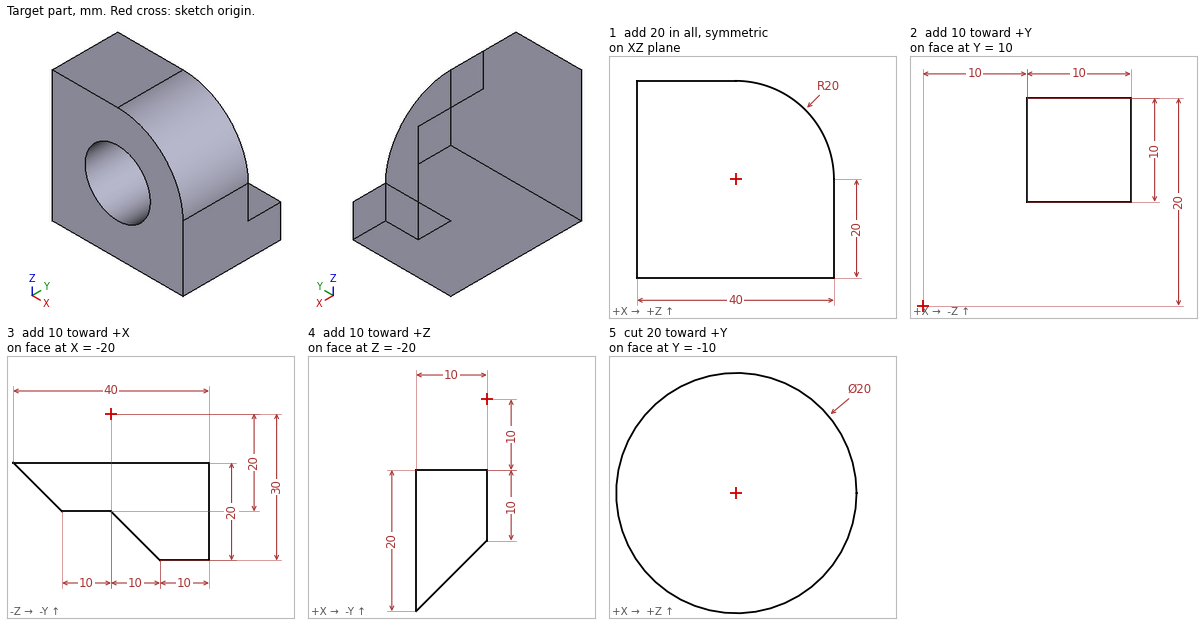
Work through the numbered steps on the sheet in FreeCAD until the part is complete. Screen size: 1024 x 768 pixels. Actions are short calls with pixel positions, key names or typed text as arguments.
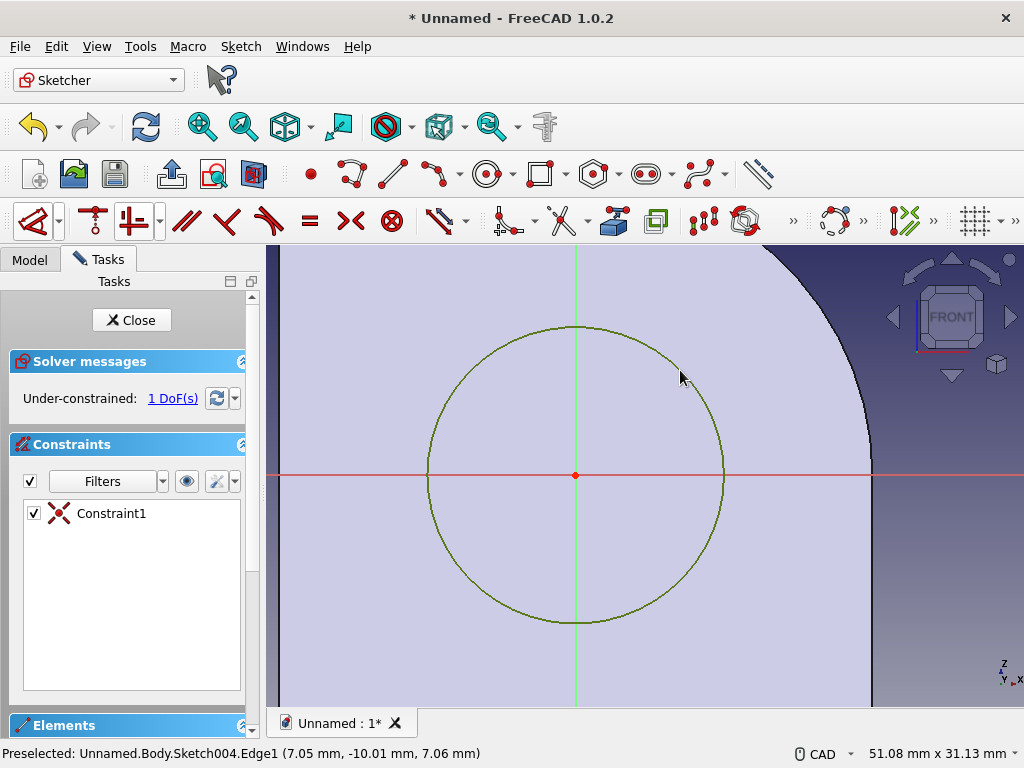
key(k)
key(o)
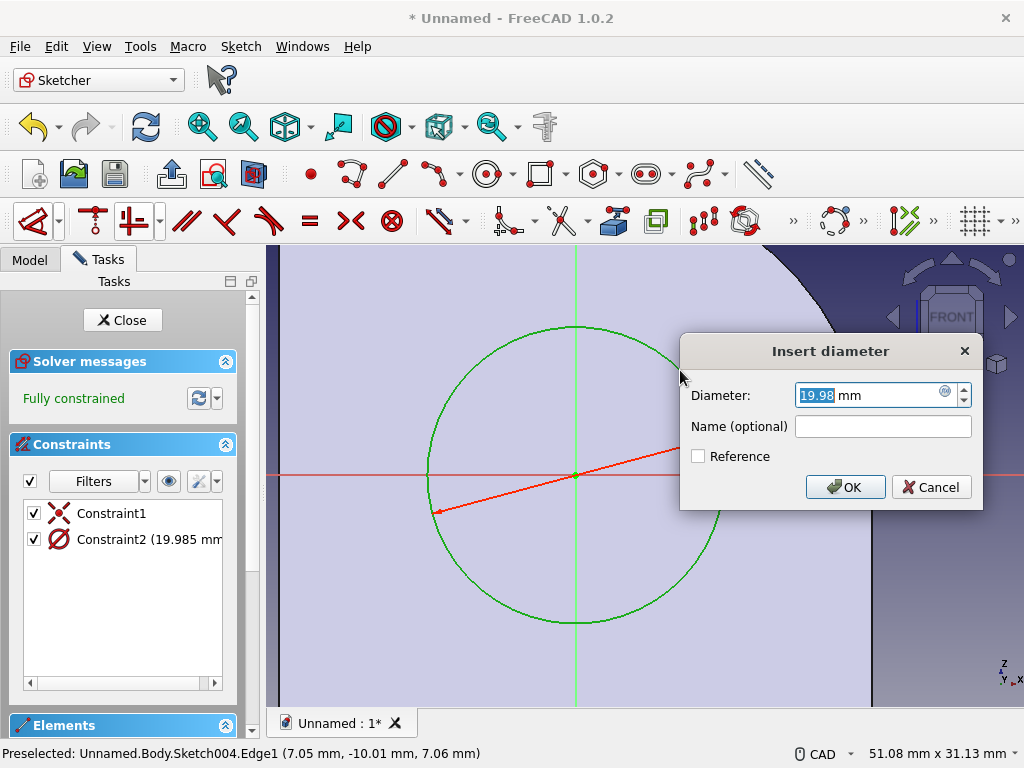
text(20)
key(Return)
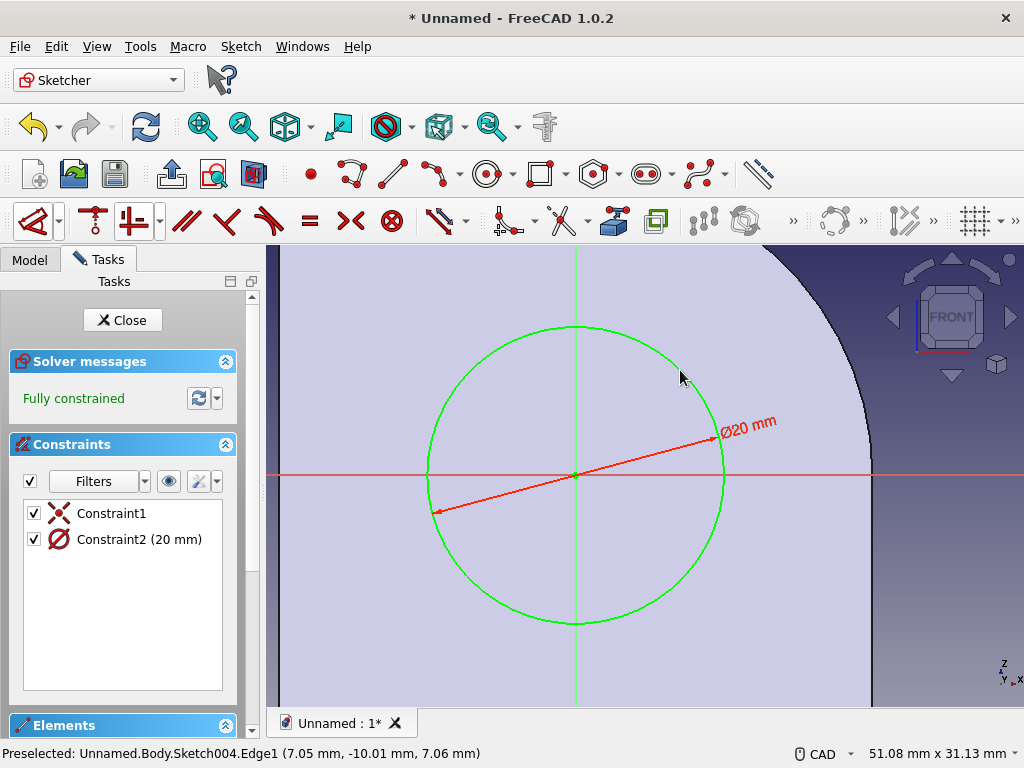
click(123, 320)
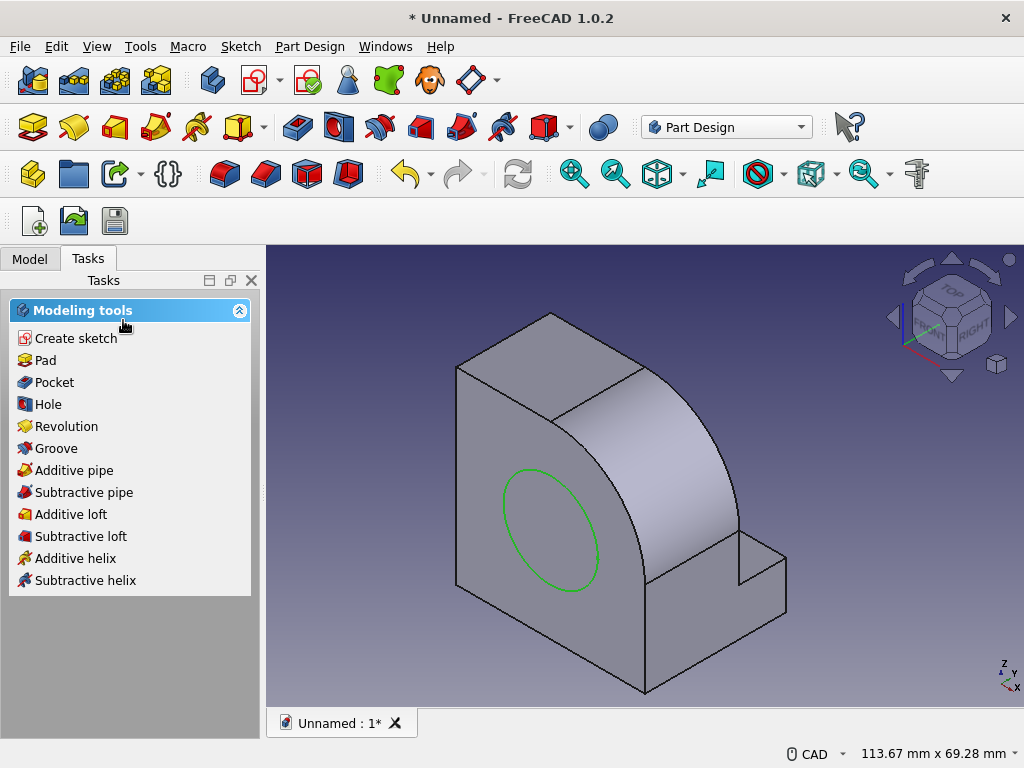
click(298, 128)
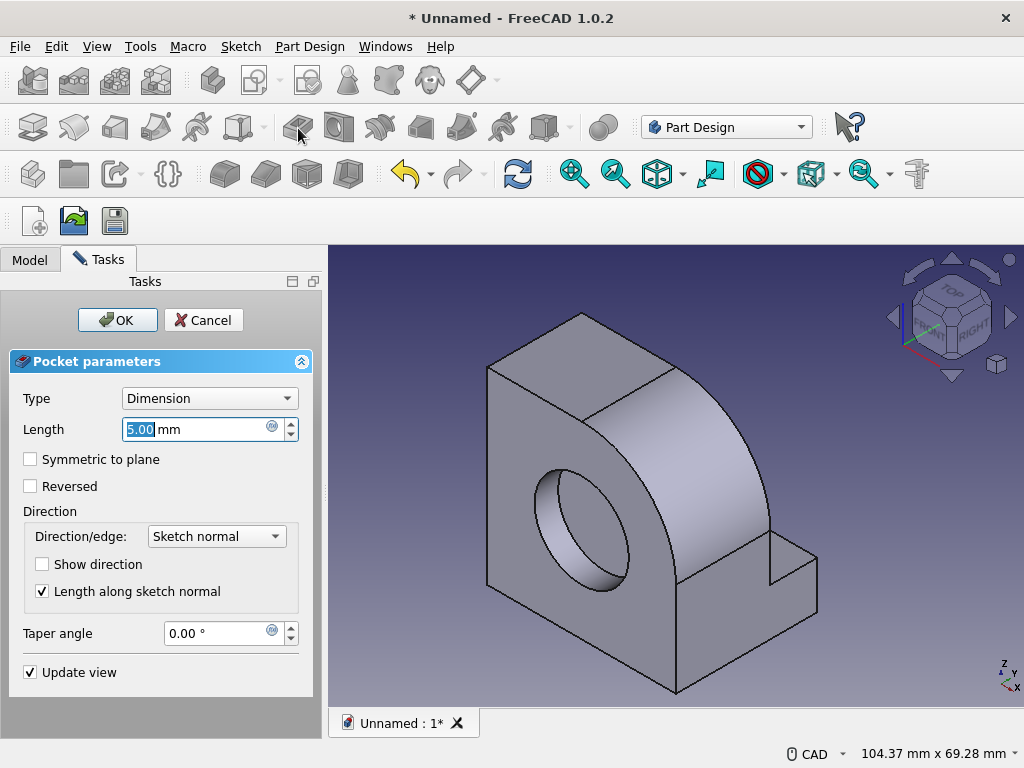
text(20)
key(Tab)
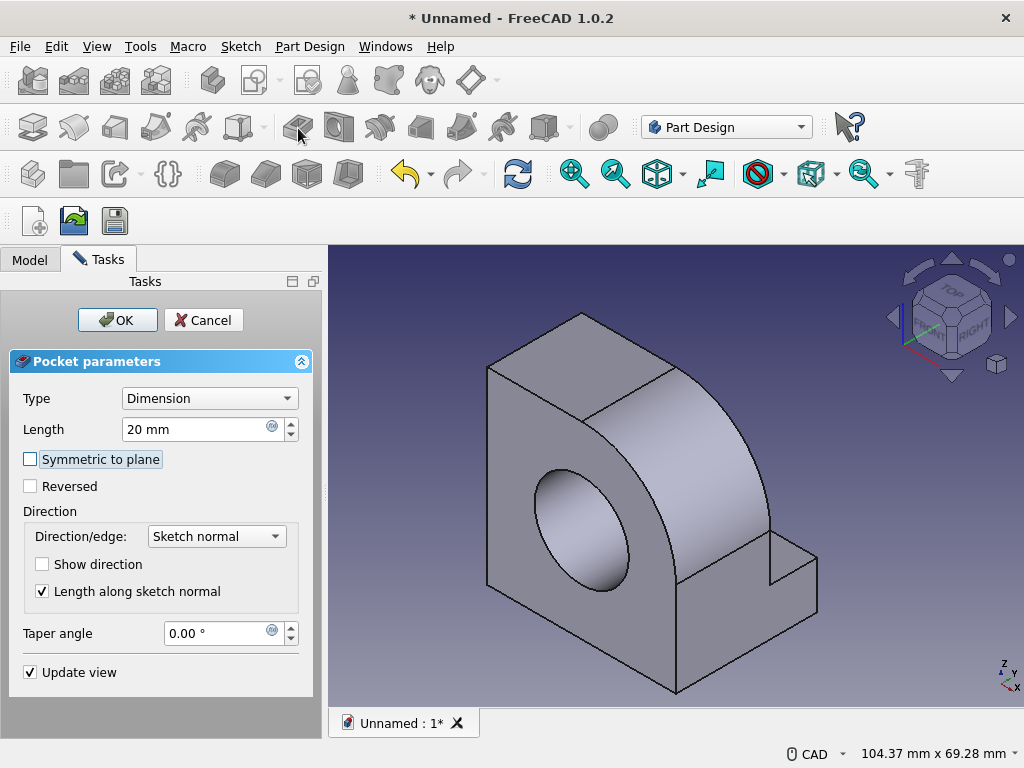
click(118, 320)